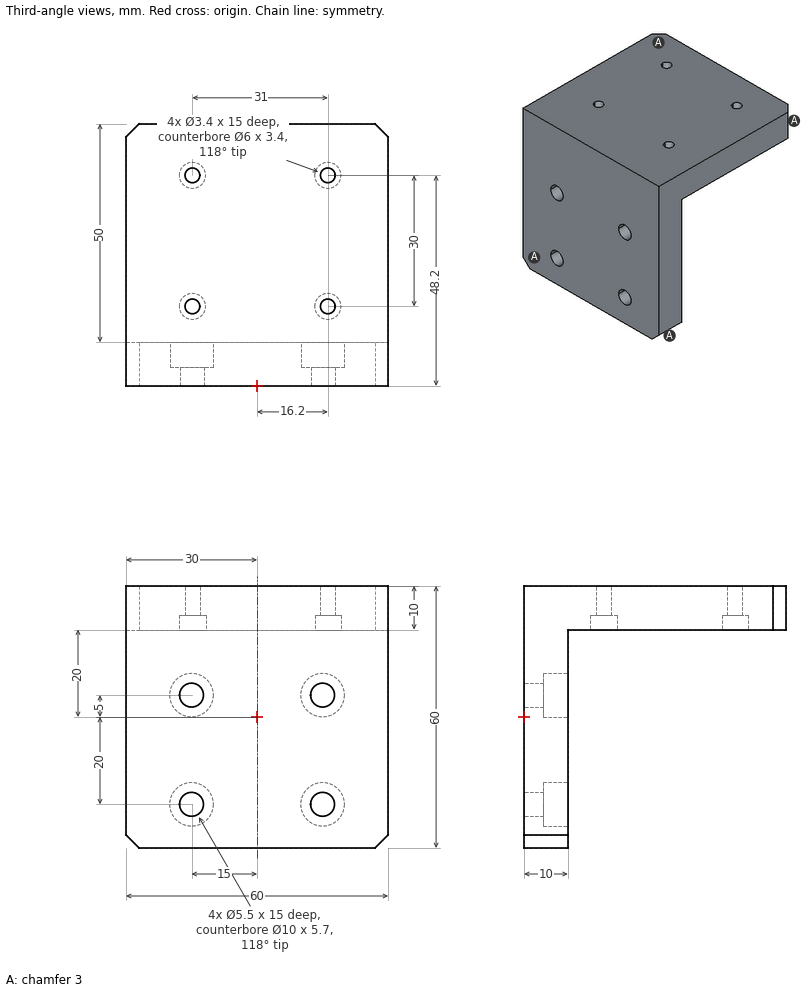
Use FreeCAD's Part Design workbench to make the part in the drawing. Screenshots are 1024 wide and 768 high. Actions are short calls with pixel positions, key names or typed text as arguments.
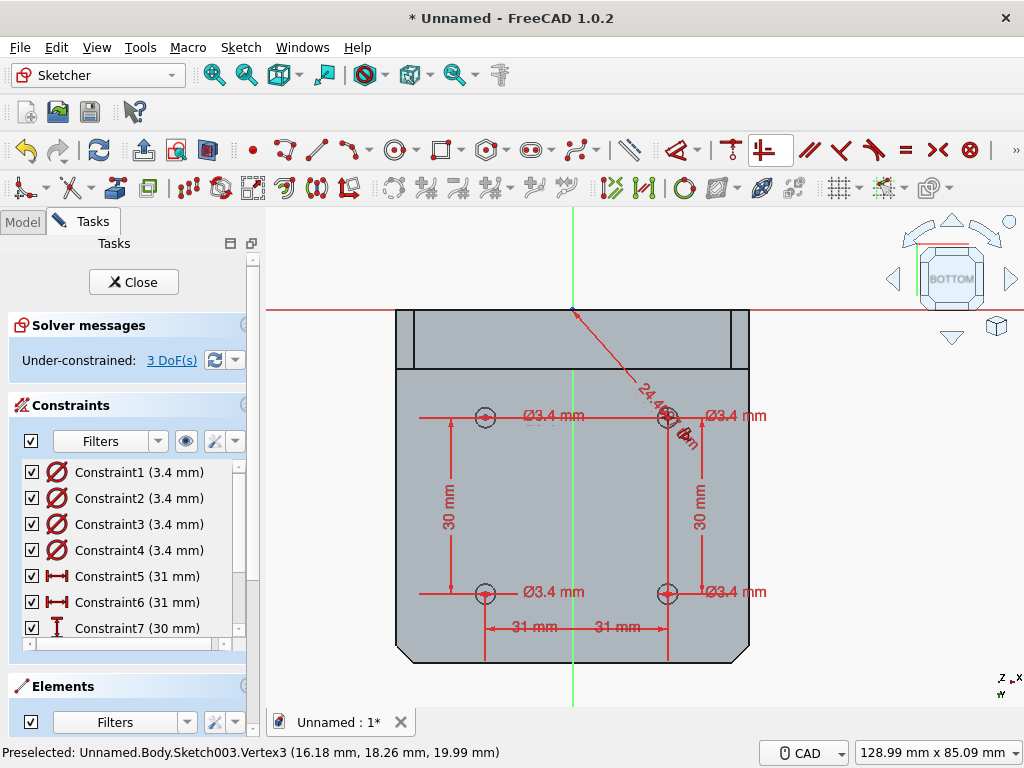
click(485, 418)
click(535, 384)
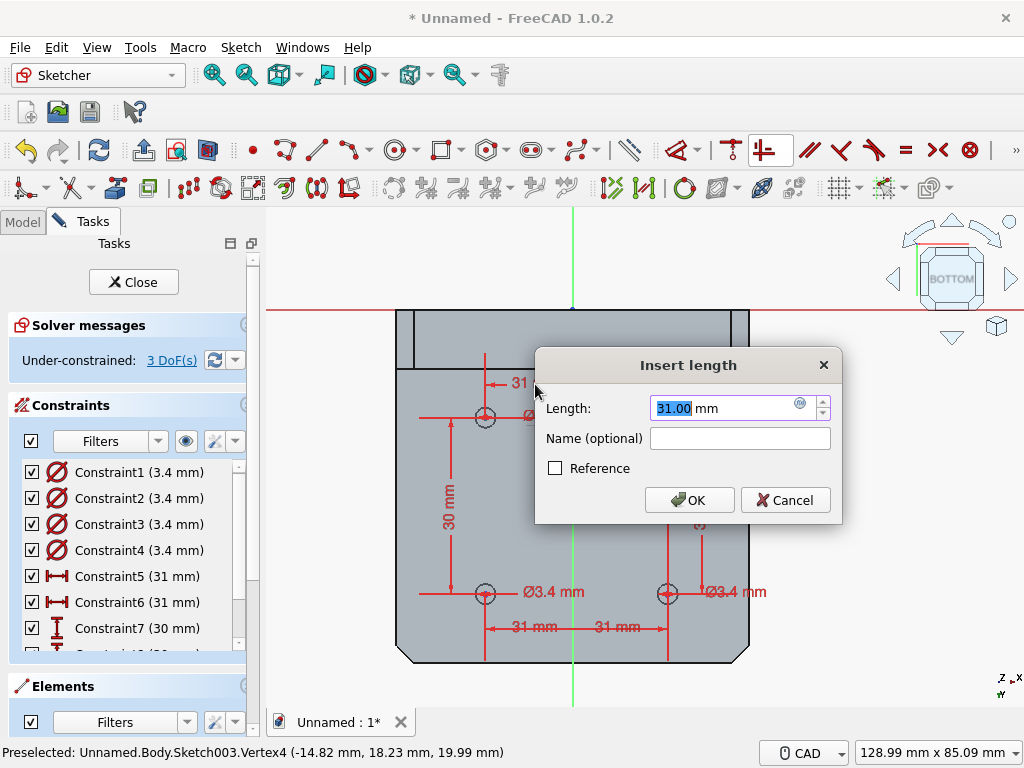
text(31)
key(Return)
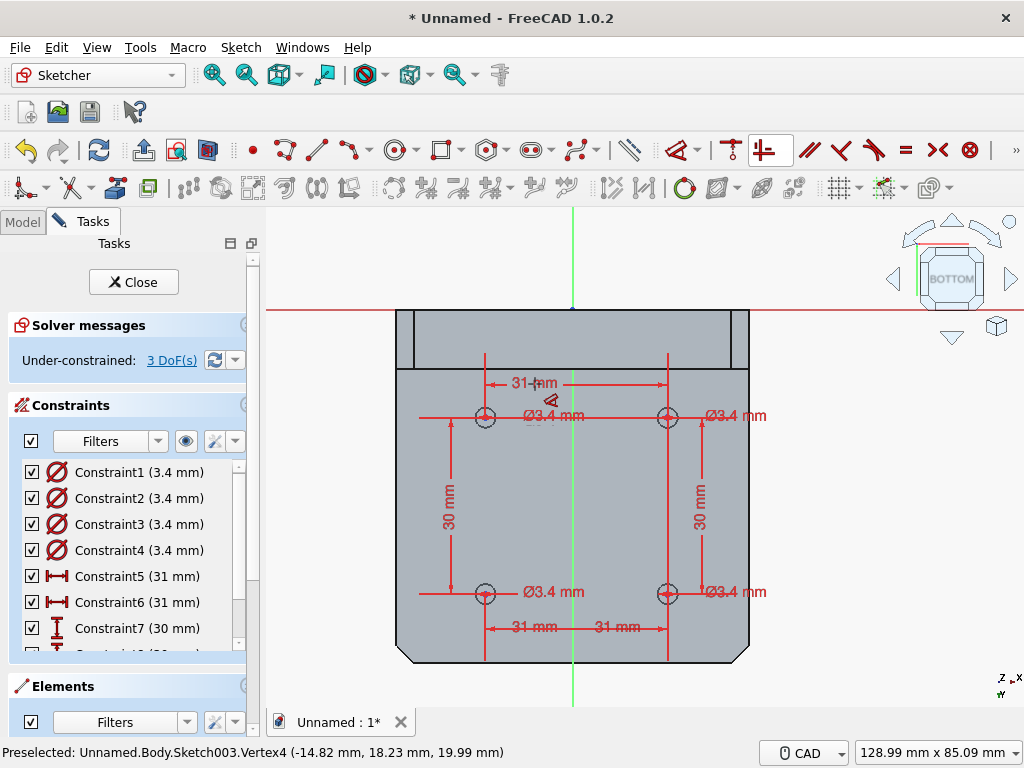
click(485, 594)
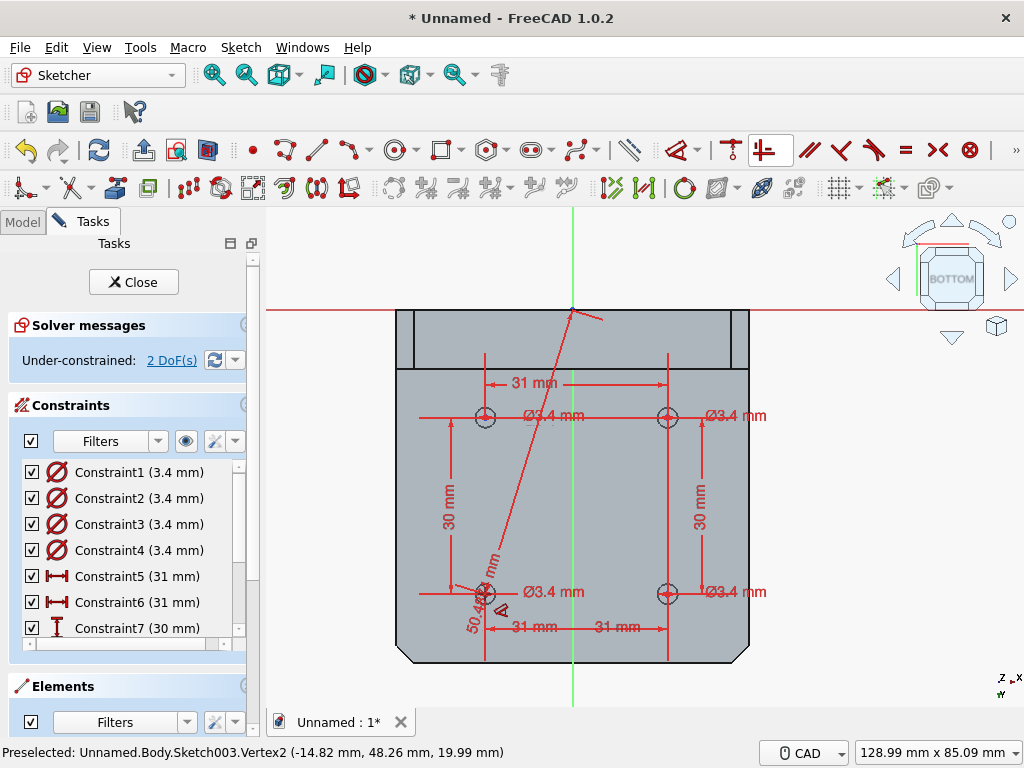
click(485, 418)
click(451, 465)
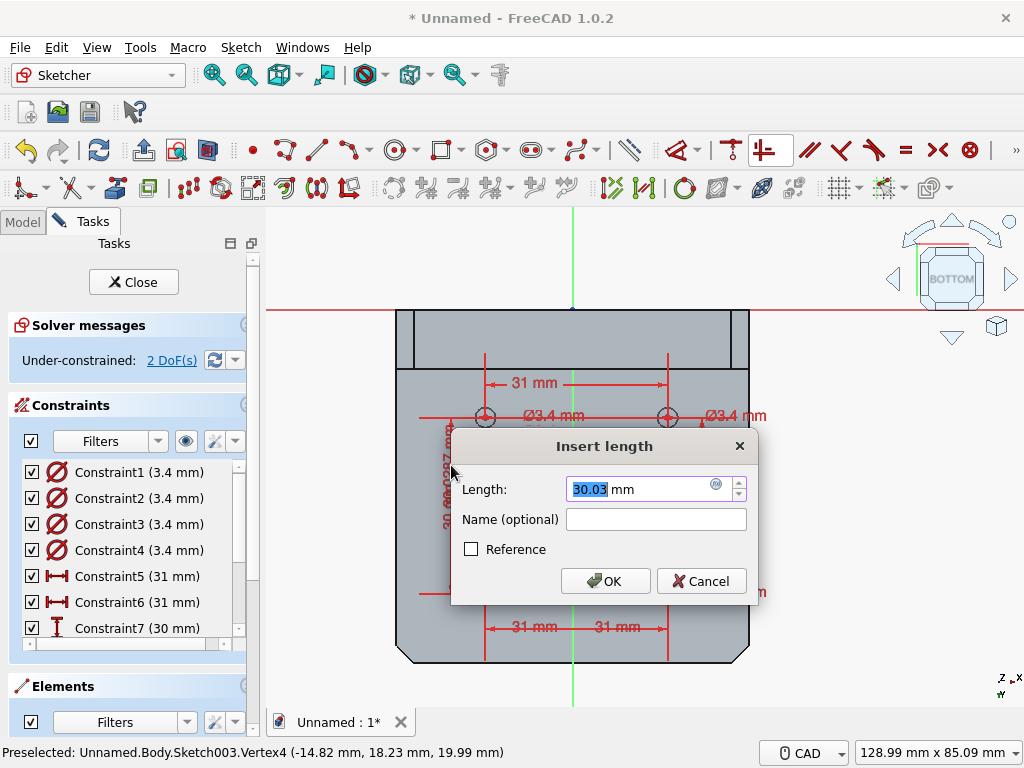
text(30)
key(Return)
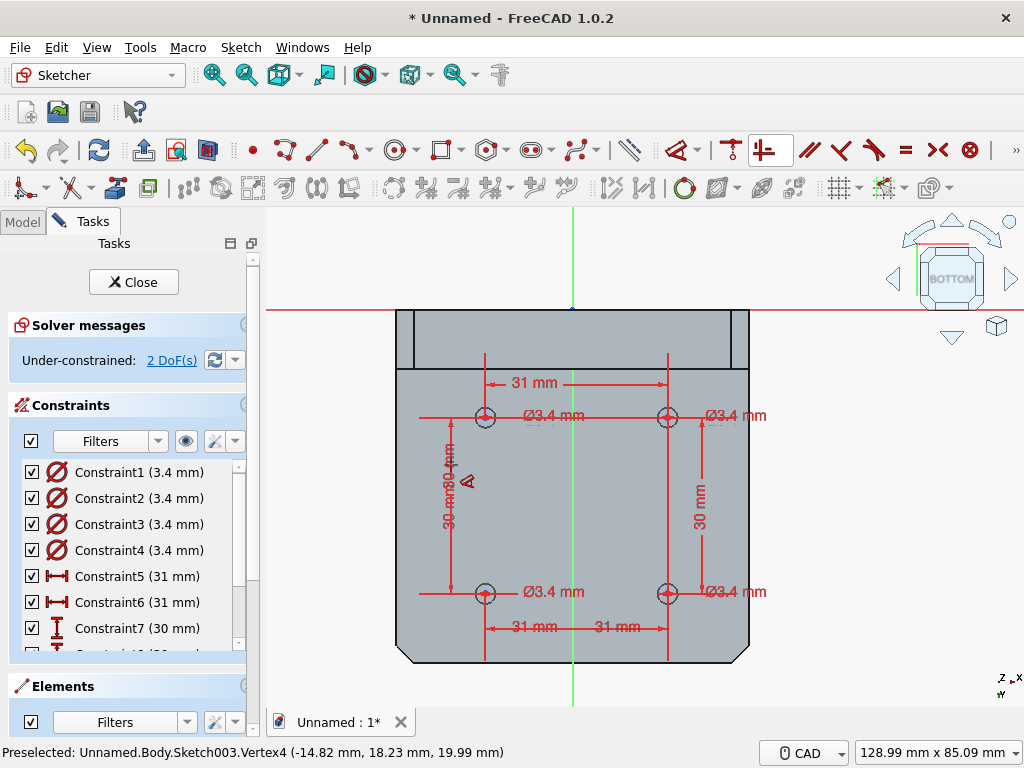
click(668, 594)
click(620, 276)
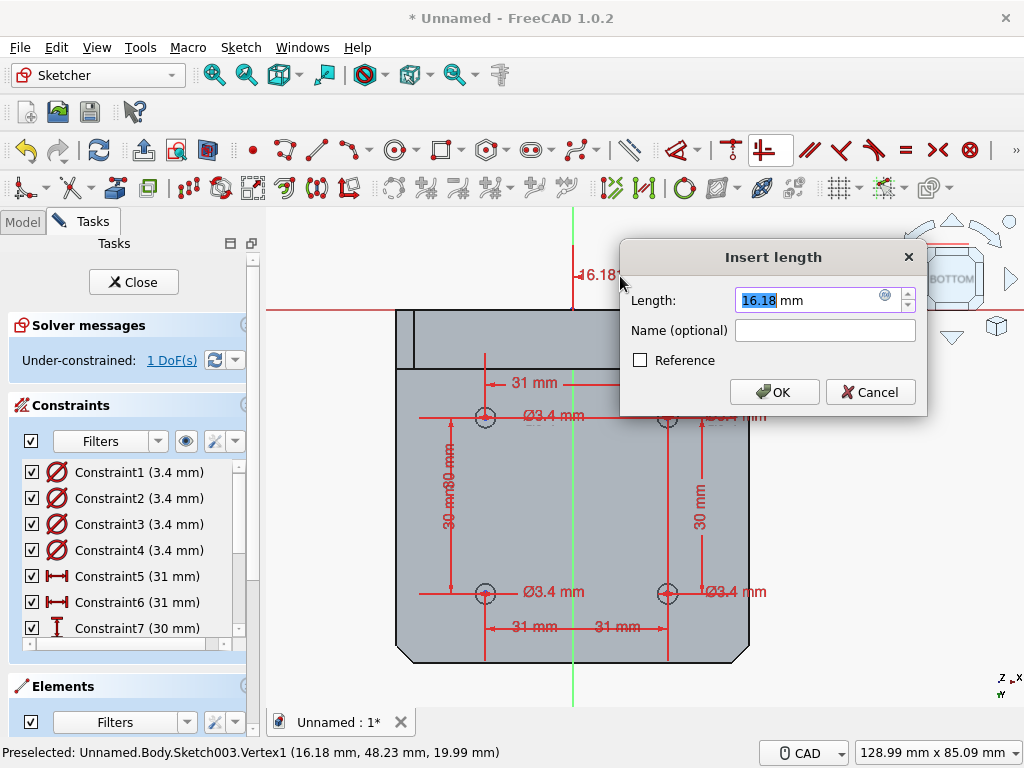
text(16.2)
key(Return)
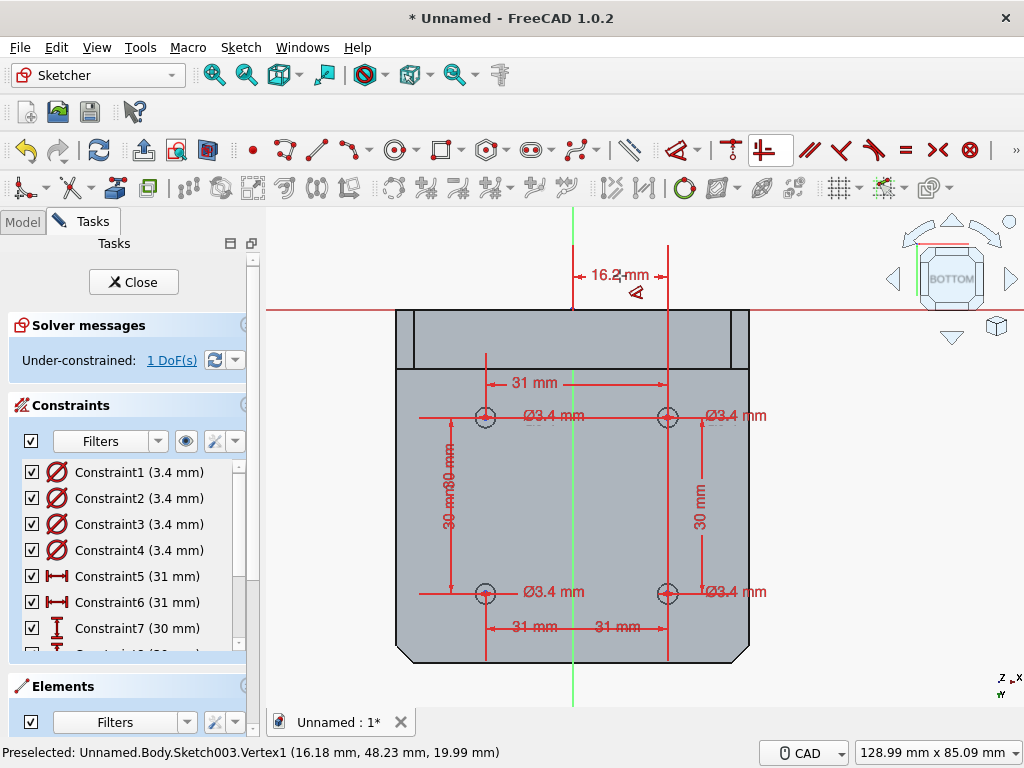
click(668, 594)
click(702, 452)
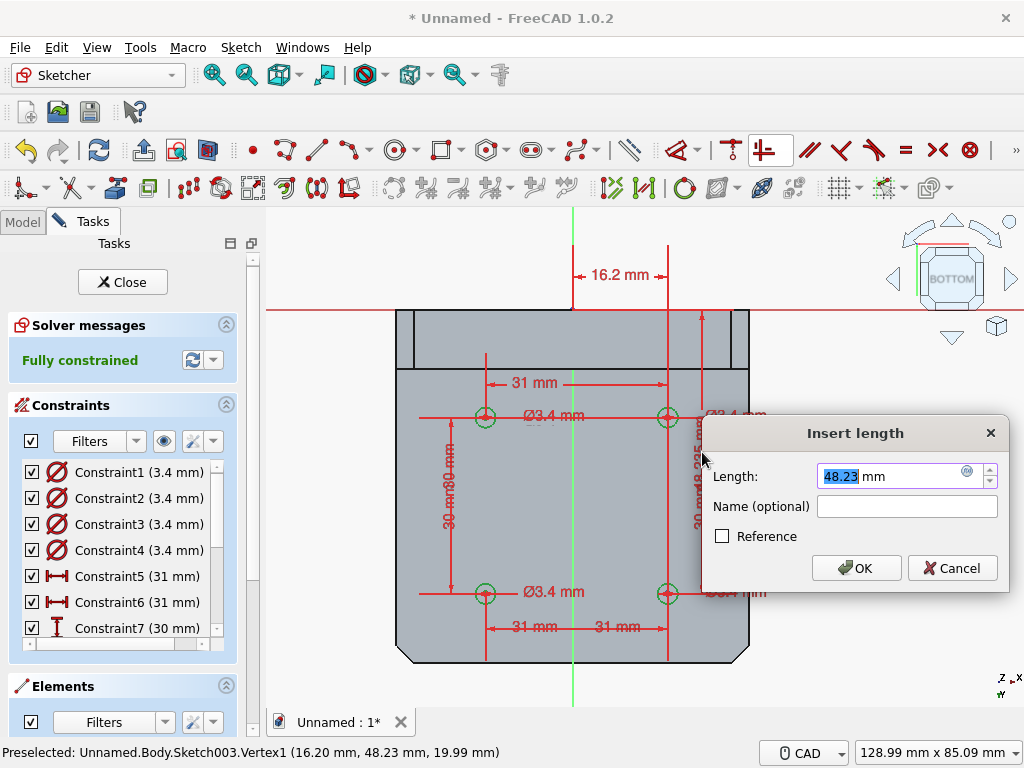
text(48.2)
key(Return)
key(Escape)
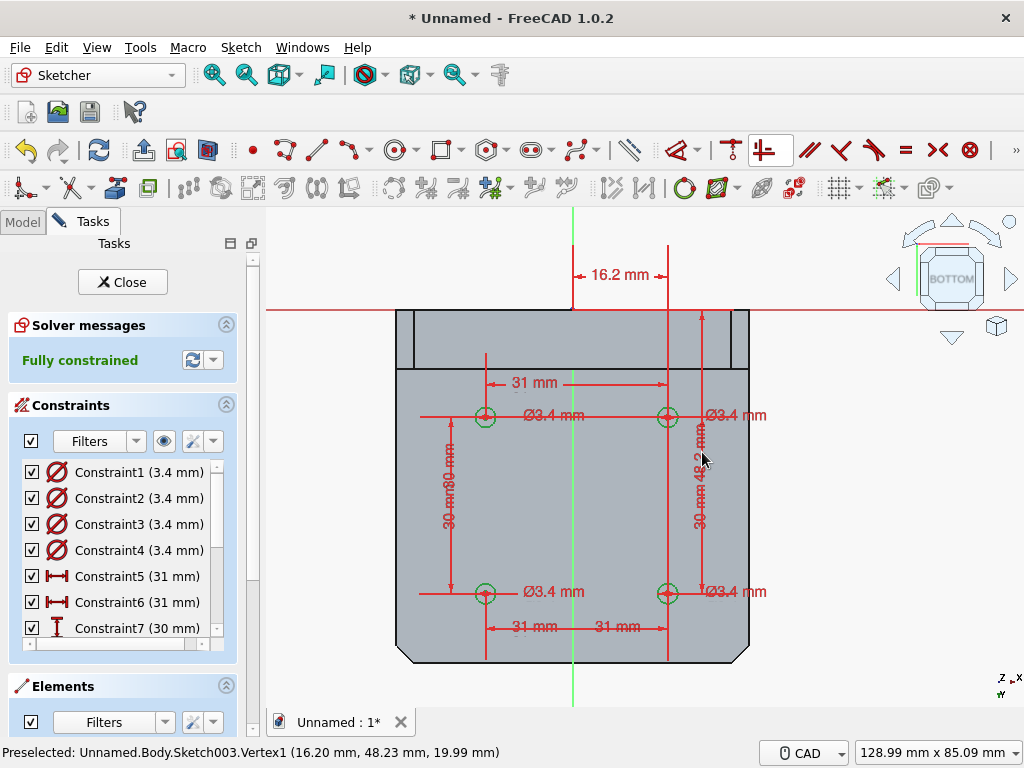
click(123, 282)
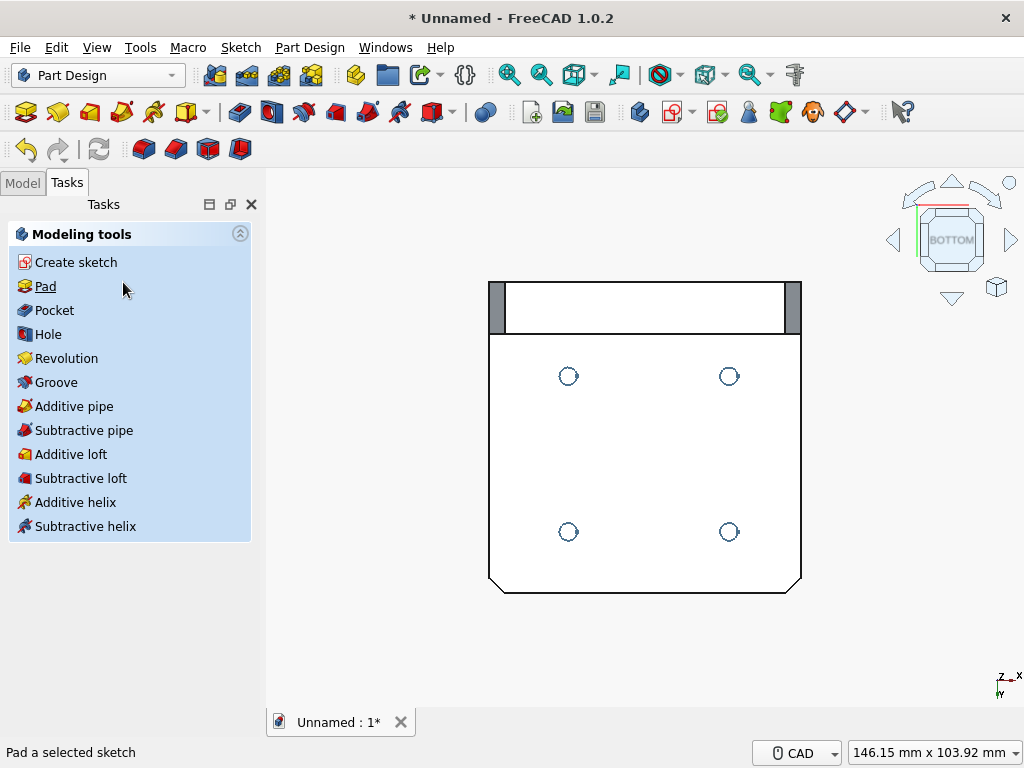
click(272, 112)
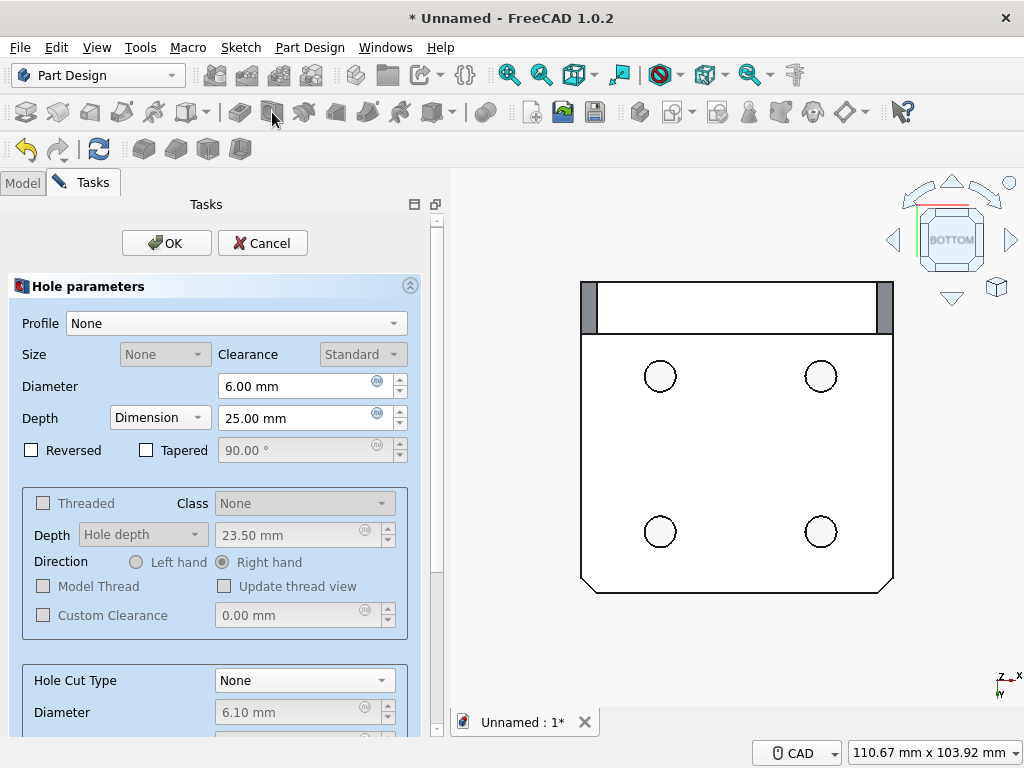
triple_click(305, 386)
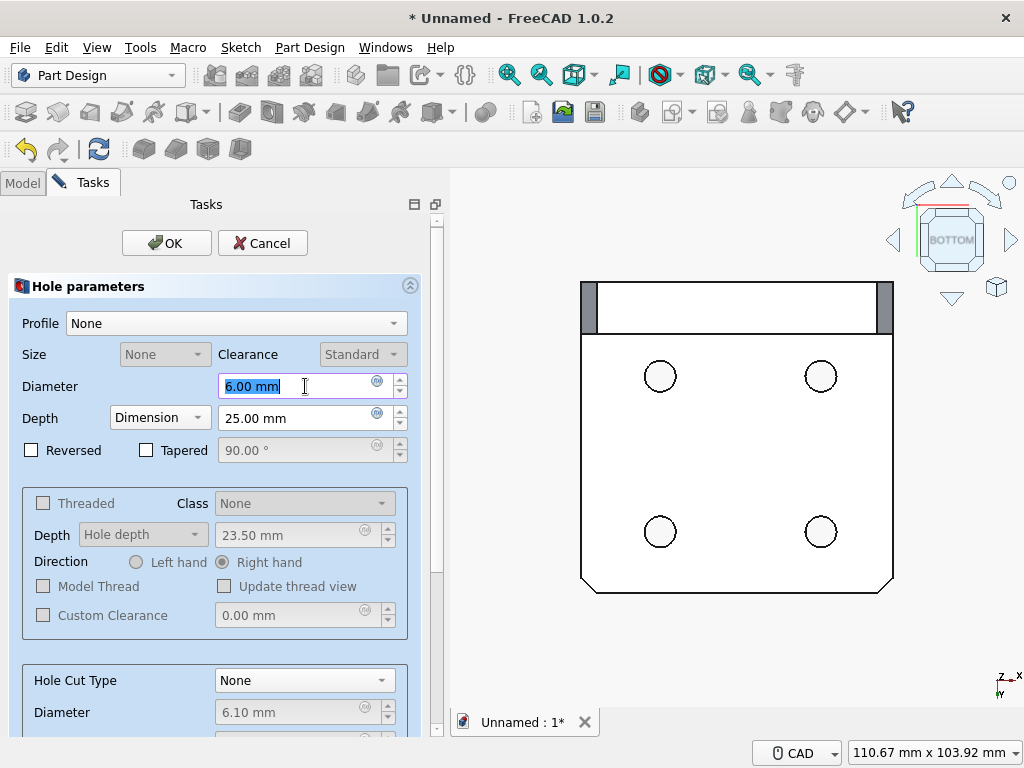
text(3.4)
key(Tab)